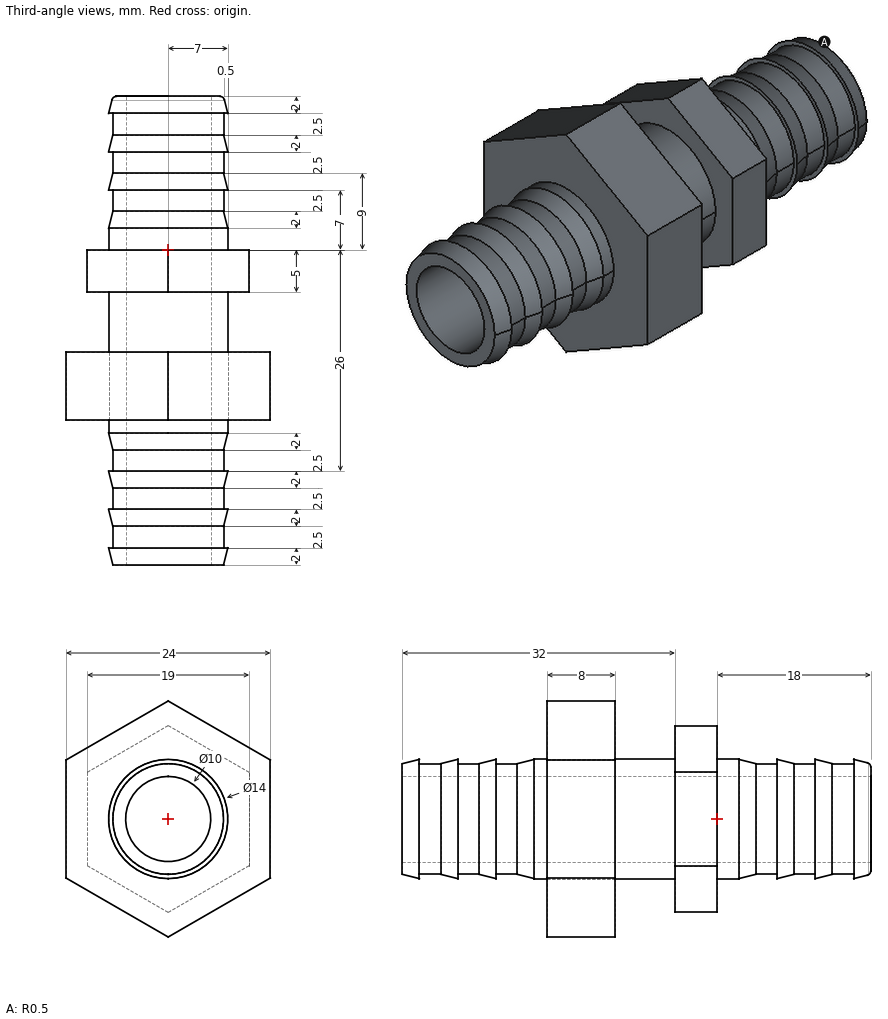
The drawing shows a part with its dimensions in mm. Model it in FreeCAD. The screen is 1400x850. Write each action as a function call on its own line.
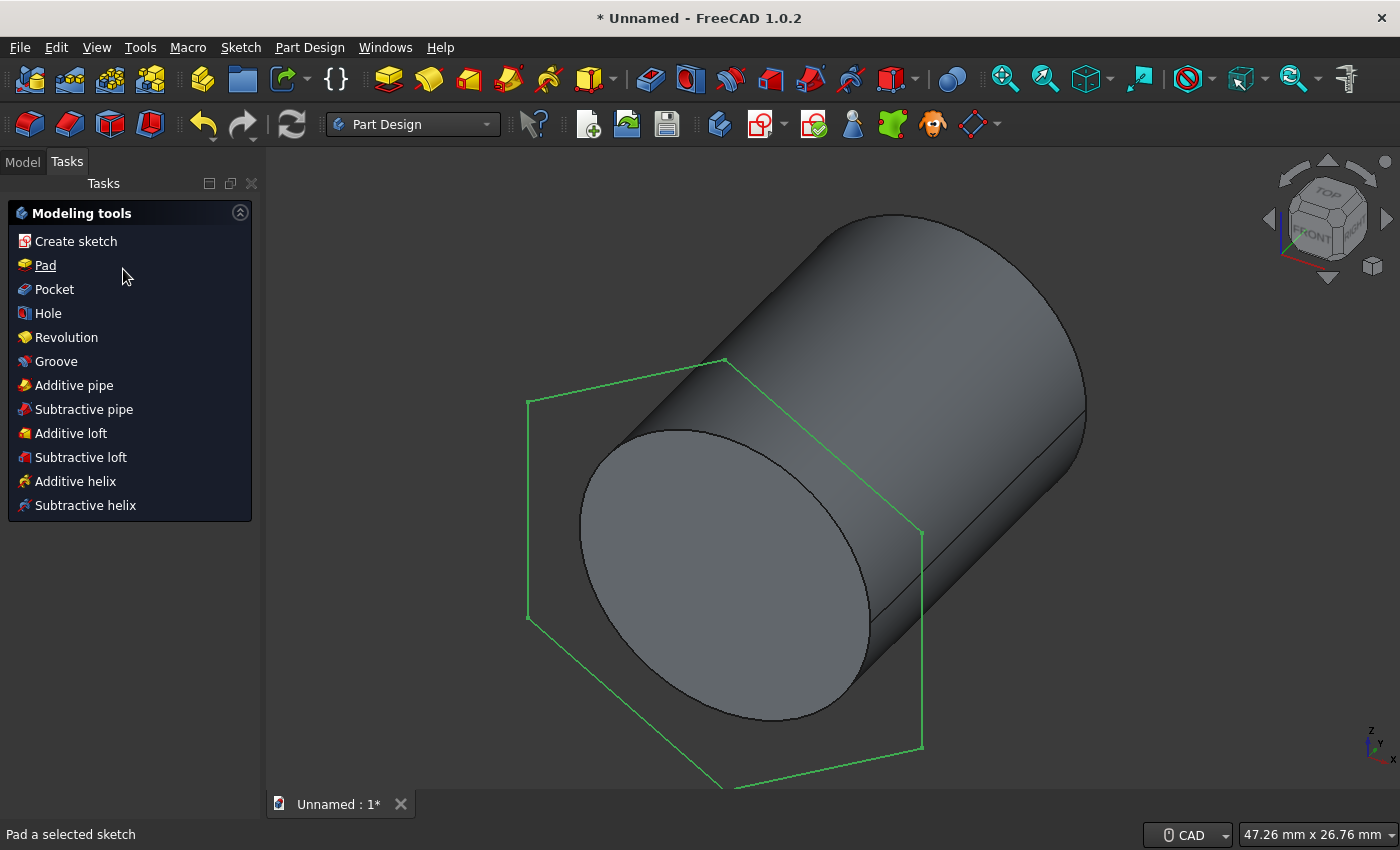
click(390, 80)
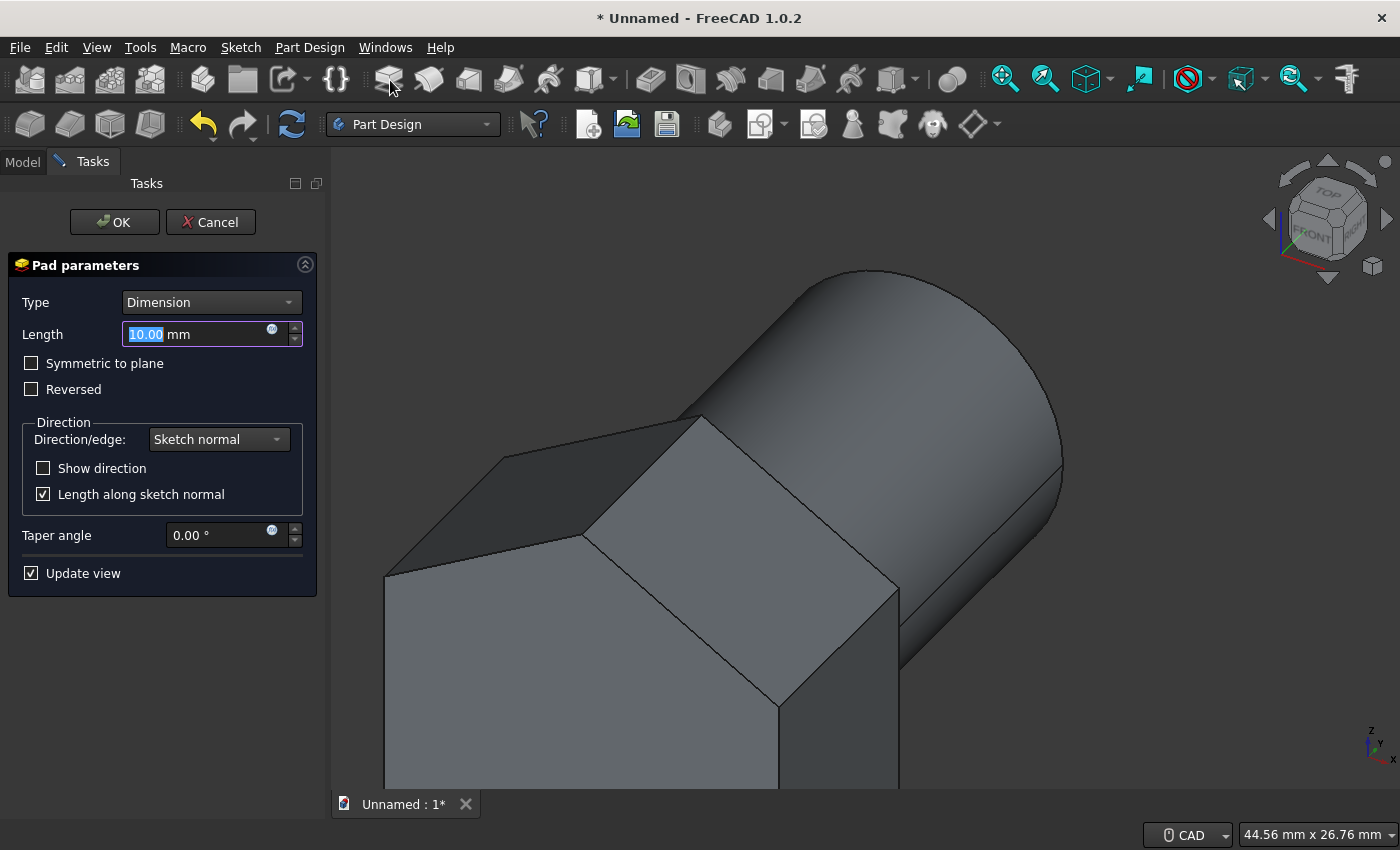
text(5)
key(Tab)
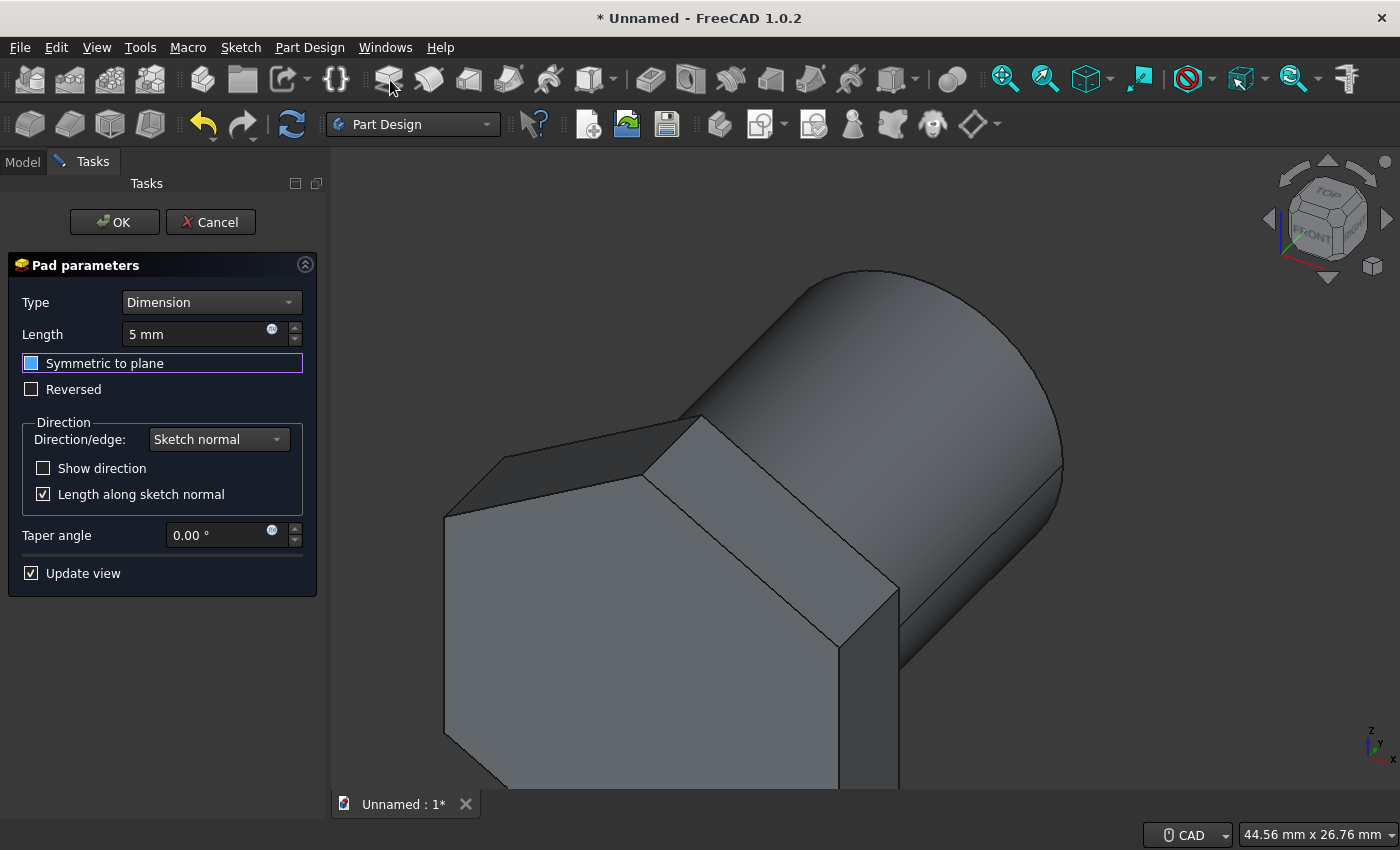
click(115, 222)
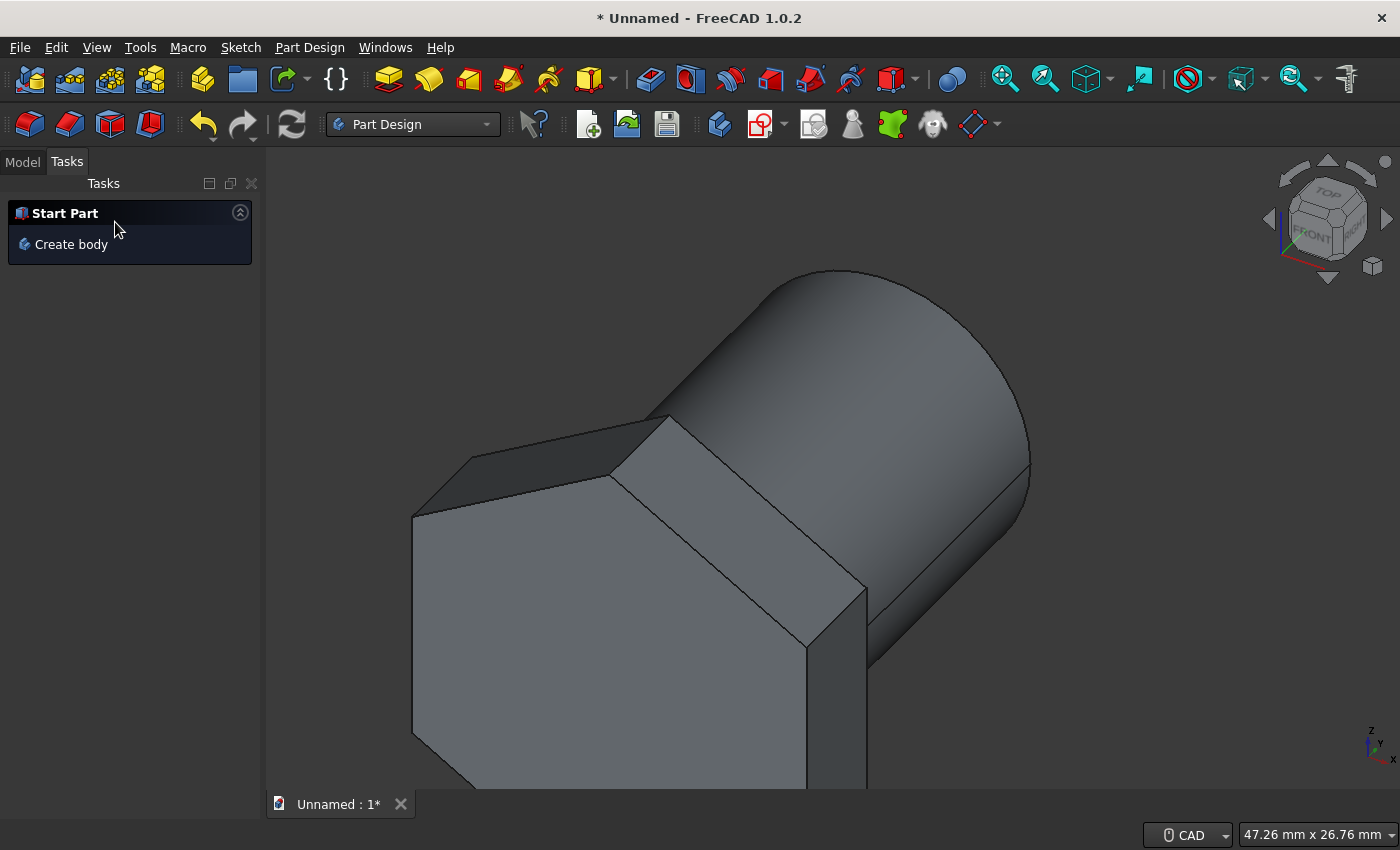
click(1006, 80)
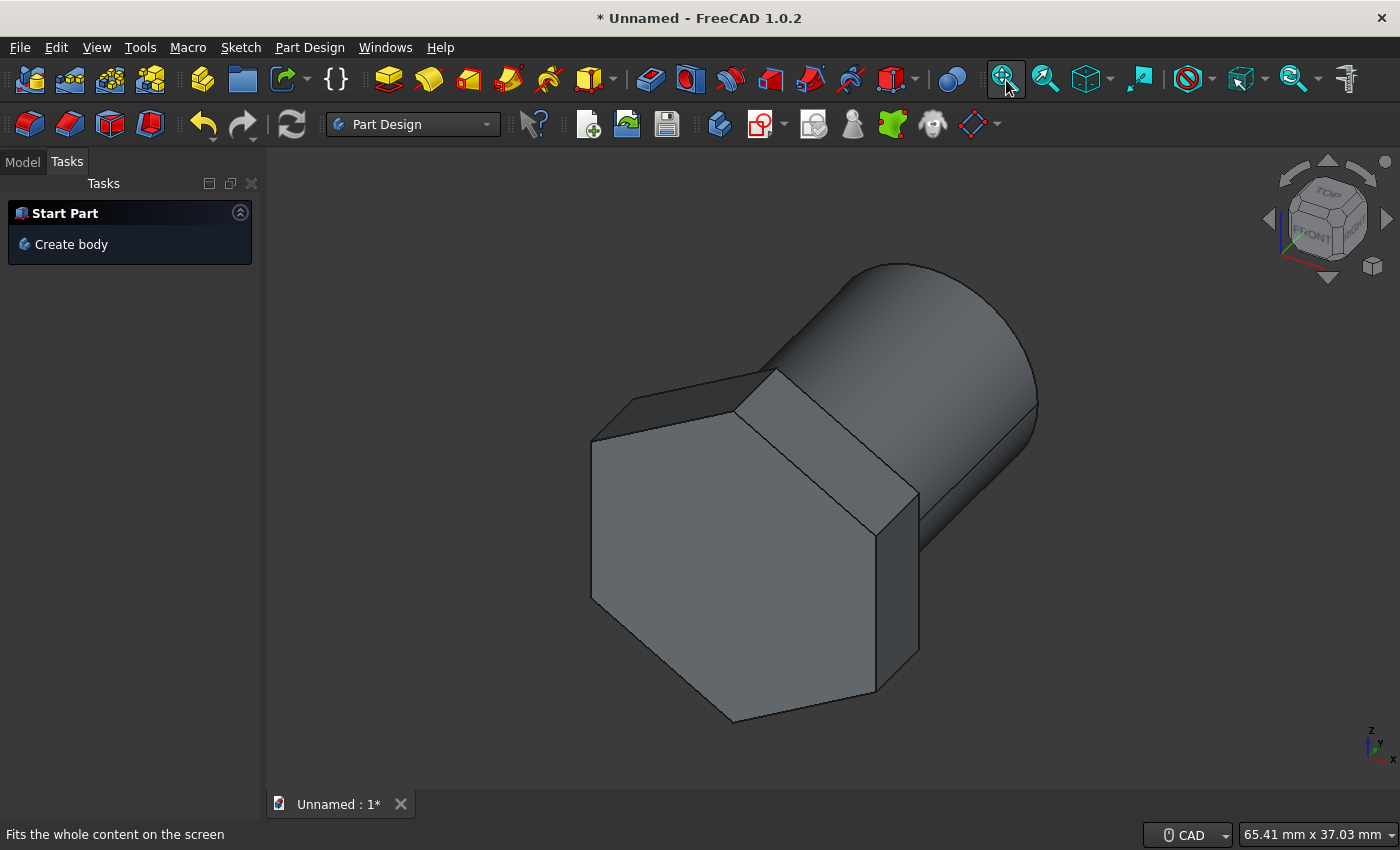
click(23, 161)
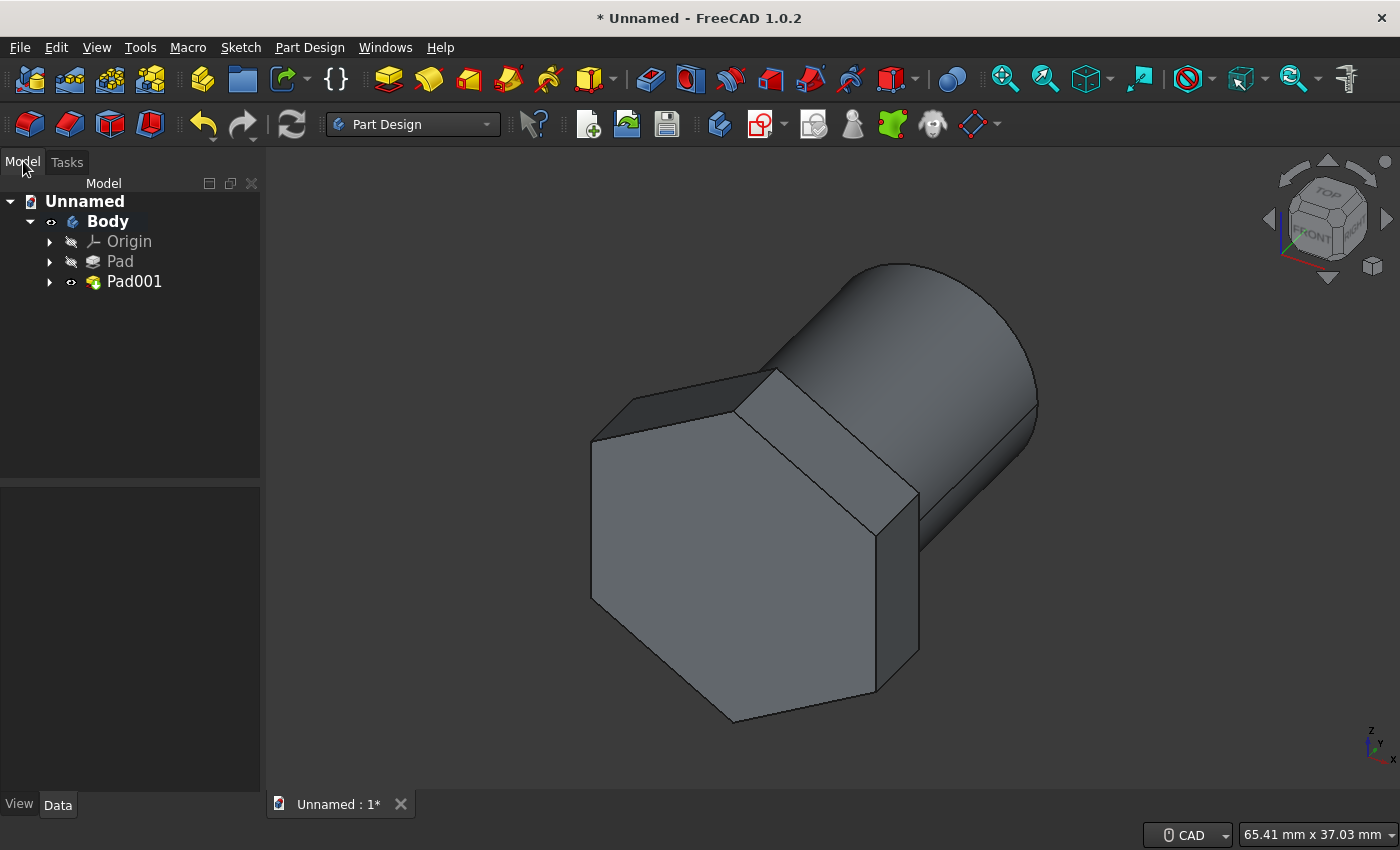
click(50, 242)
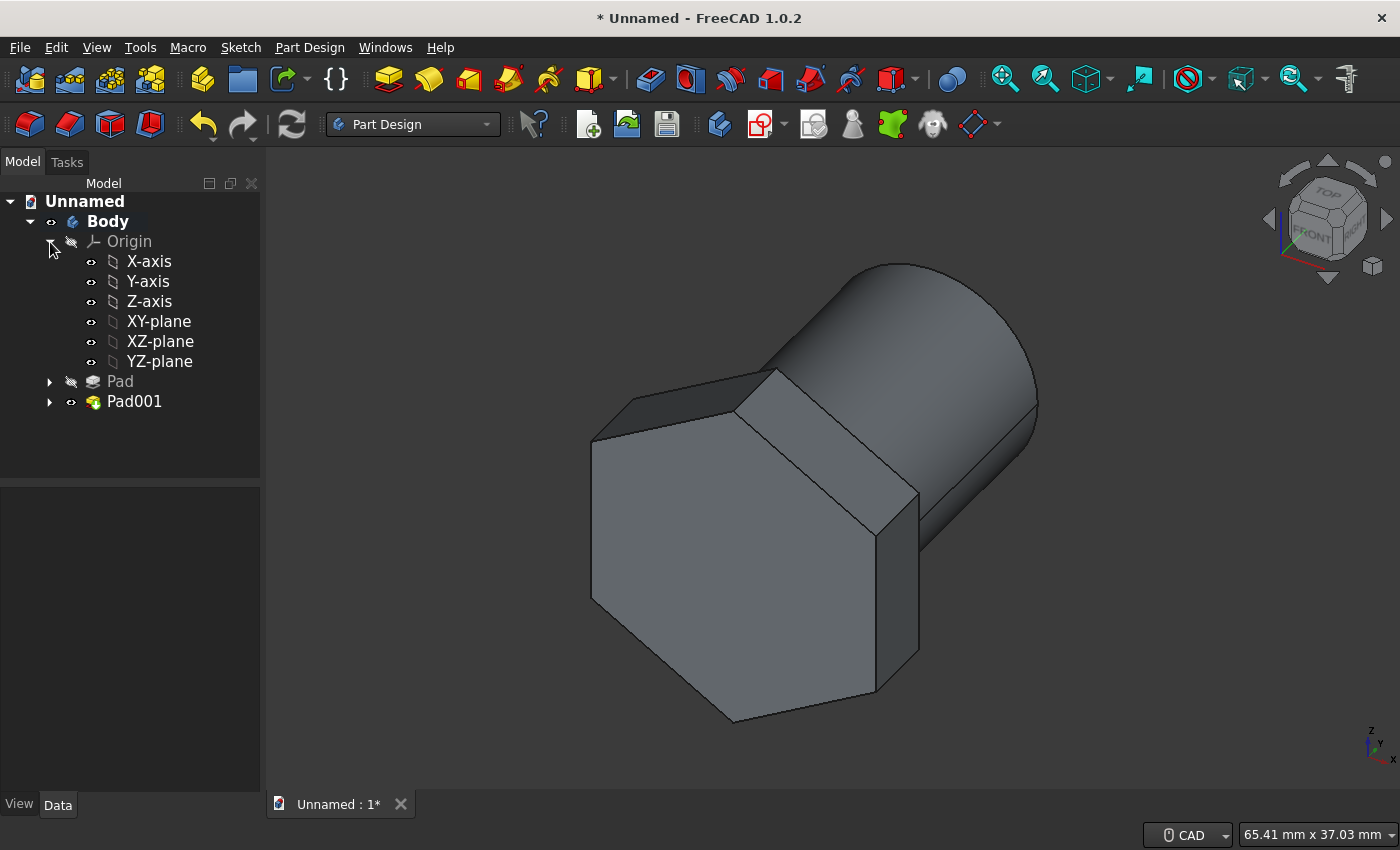
click(136, 342)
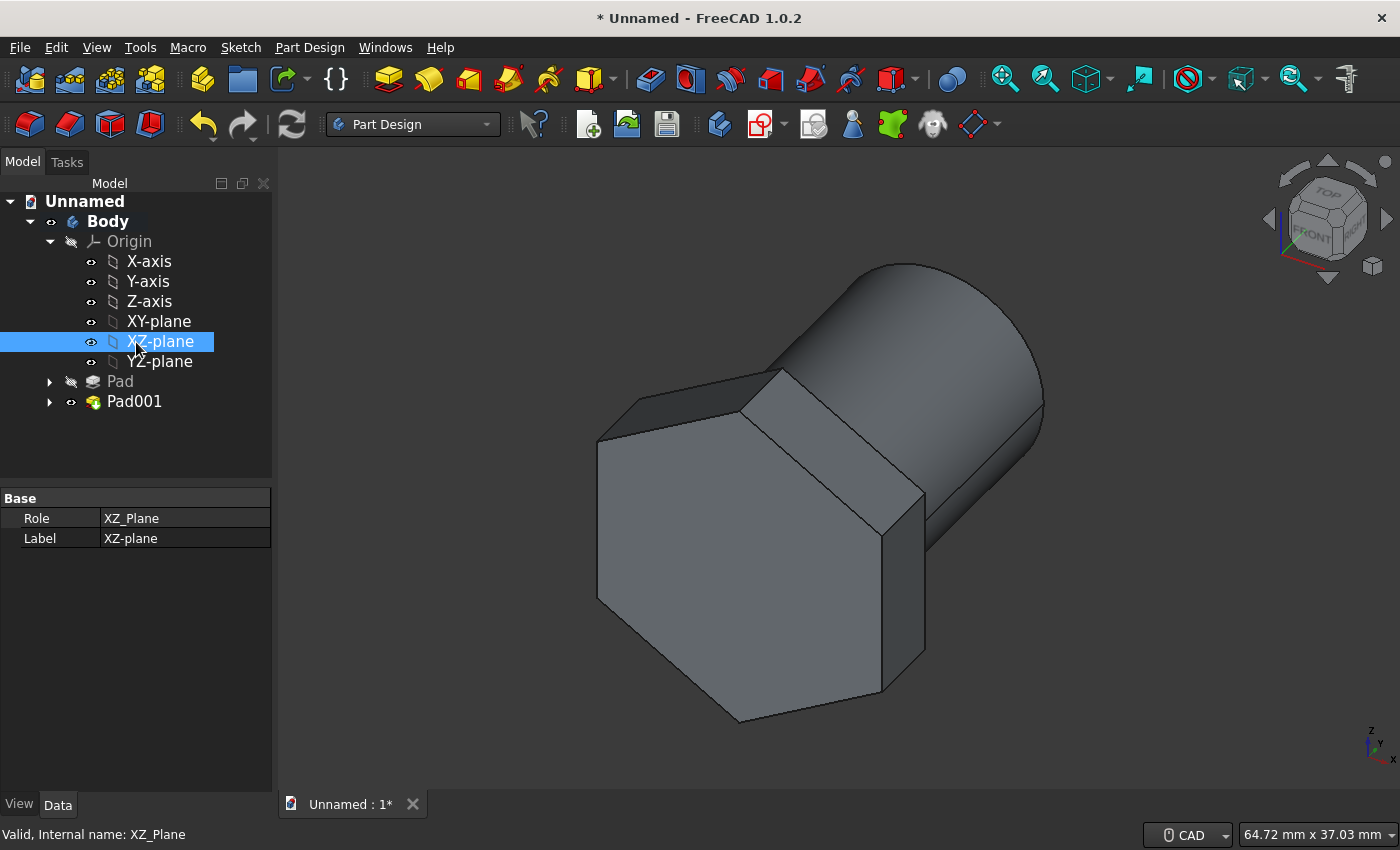
click(974, 124)